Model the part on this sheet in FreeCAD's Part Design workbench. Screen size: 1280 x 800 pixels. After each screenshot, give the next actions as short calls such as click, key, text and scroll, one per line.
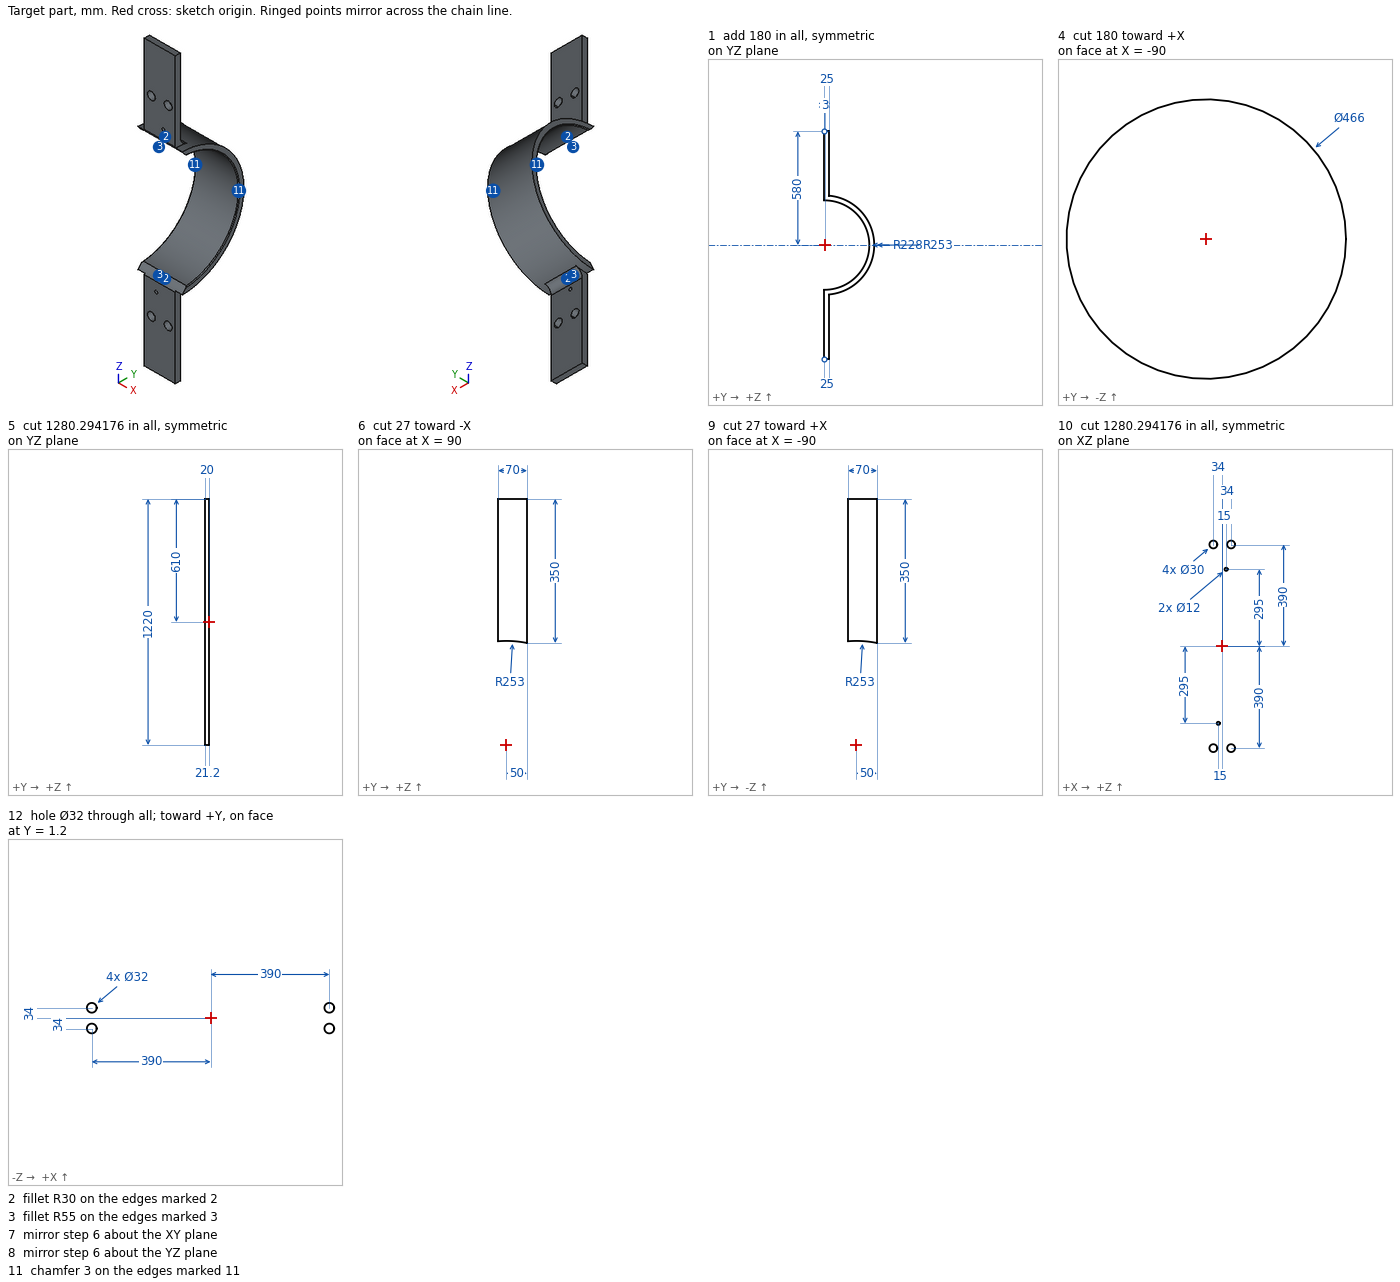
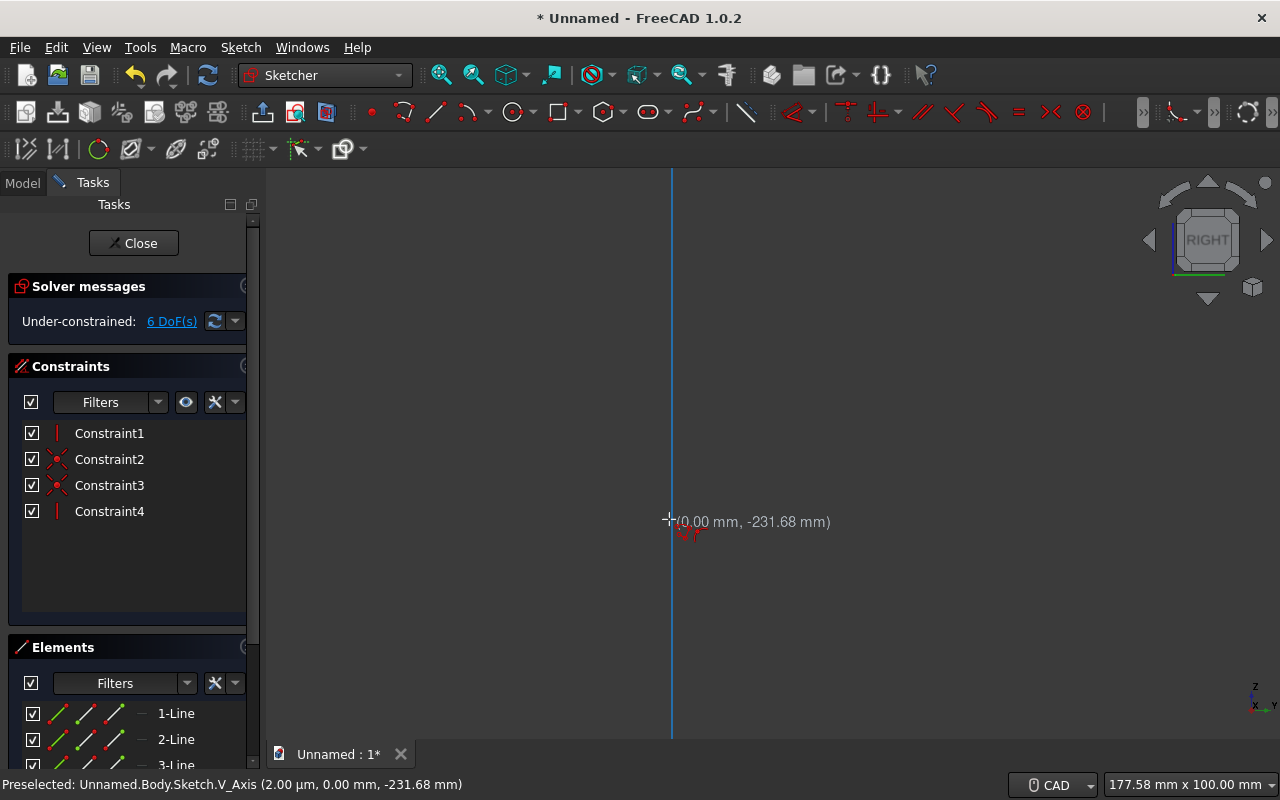
click(655, 506)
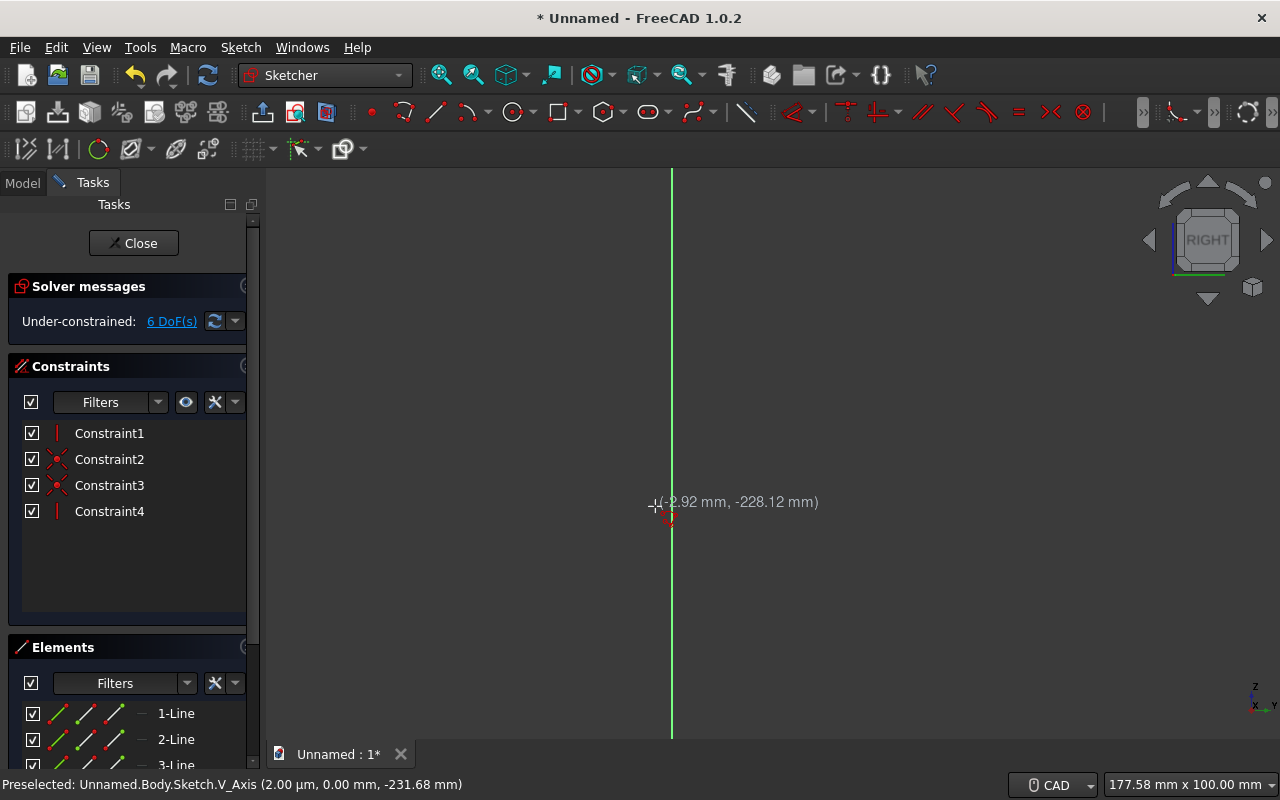
scroll(669, 519, down, 15)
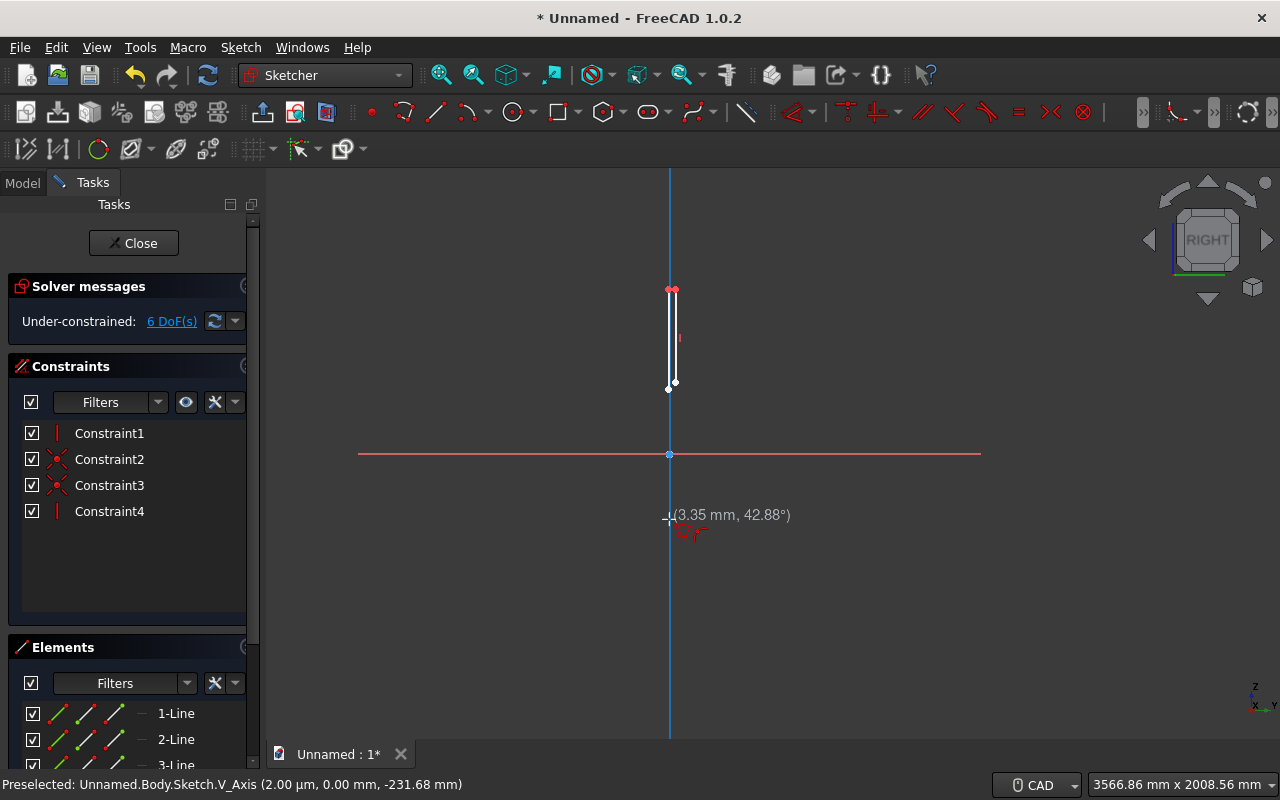
scroll(669, 619, up, 15)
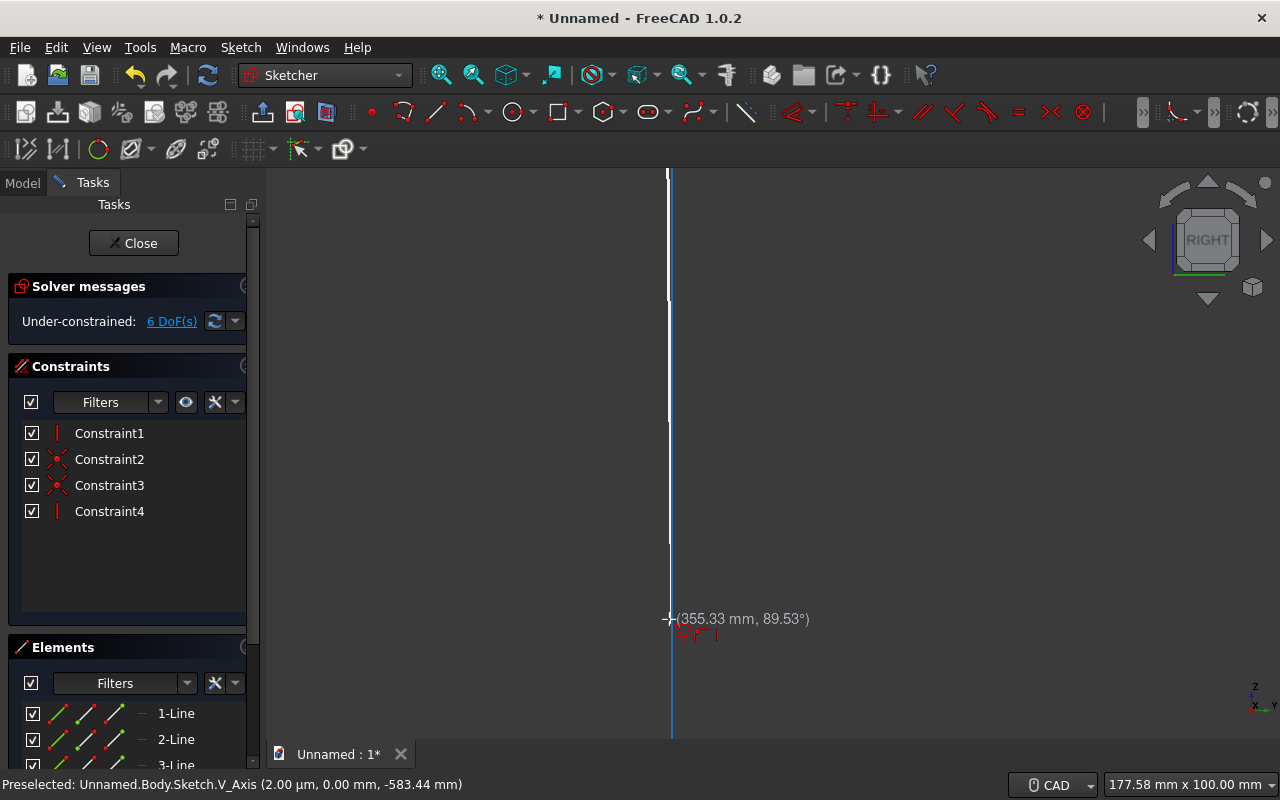
click(655, 604)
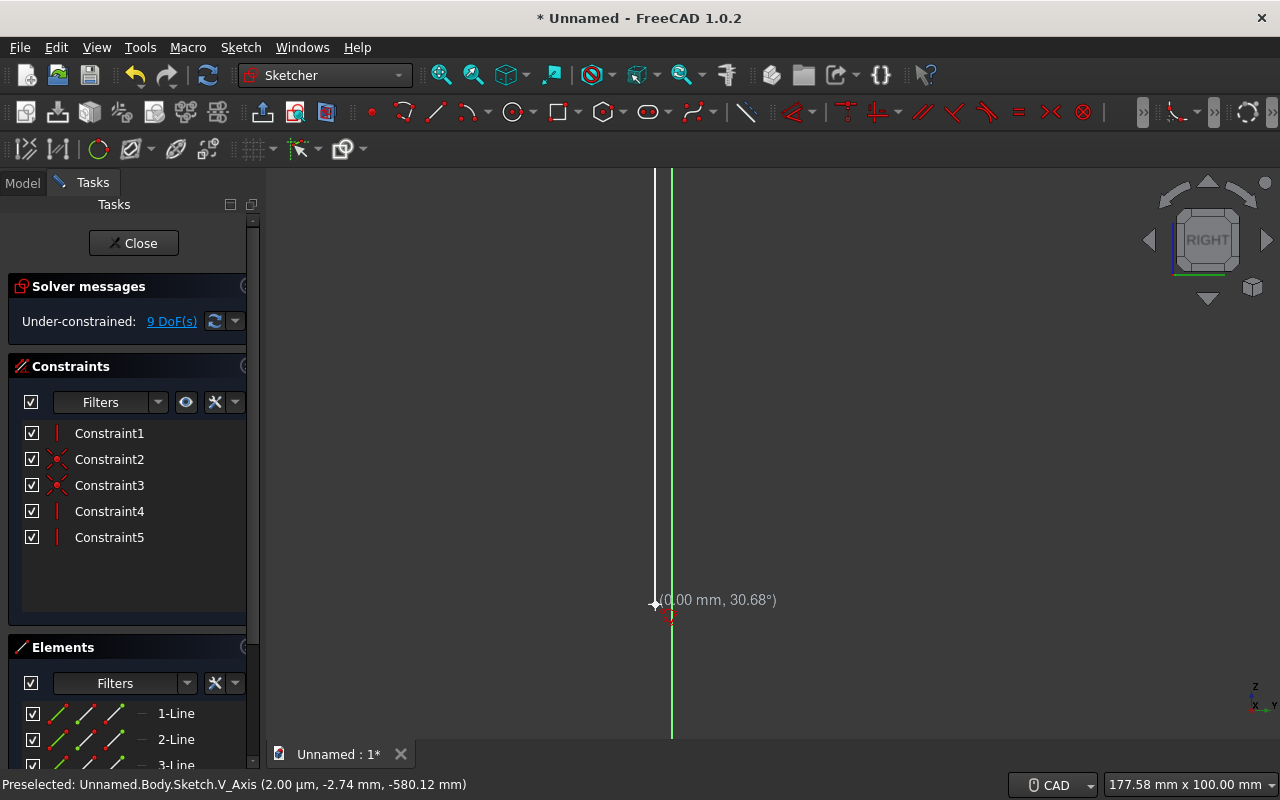
scroll(669, 619, down, 15)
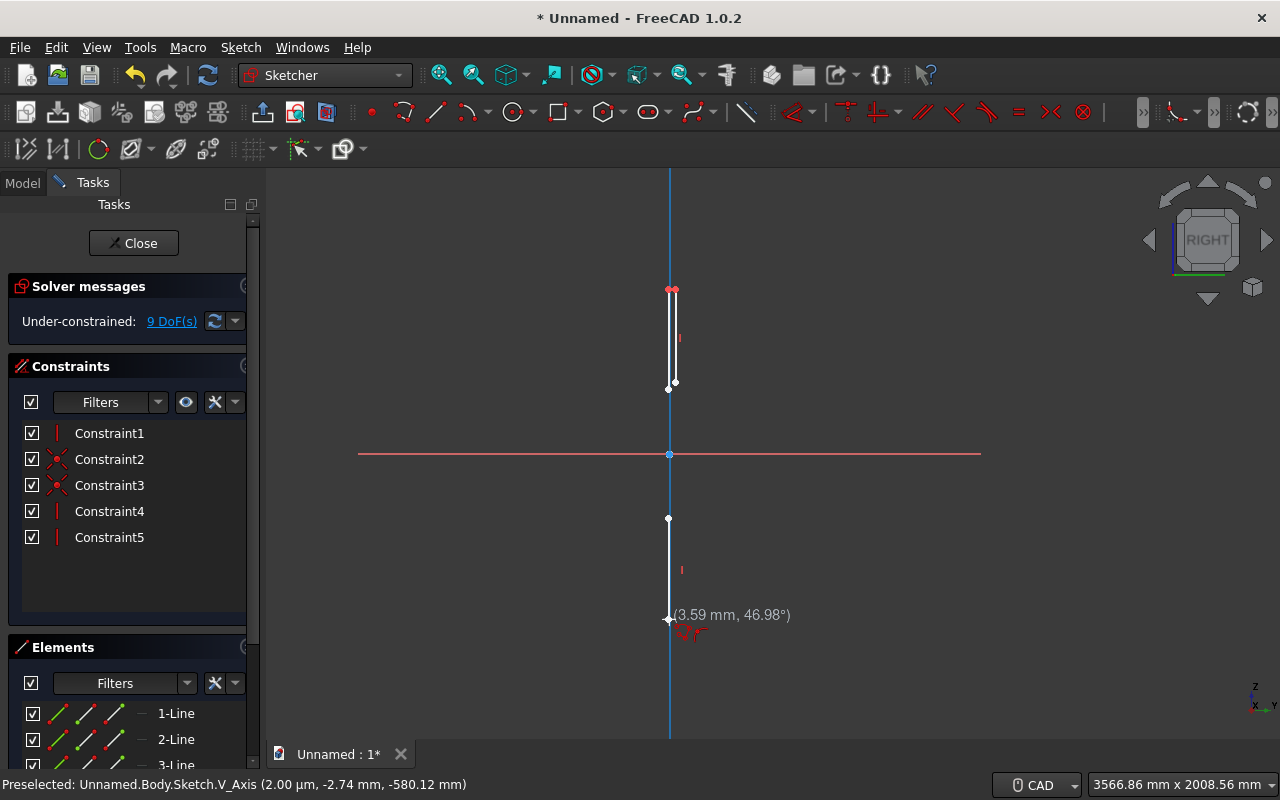
scroll(676, 619, up, 5)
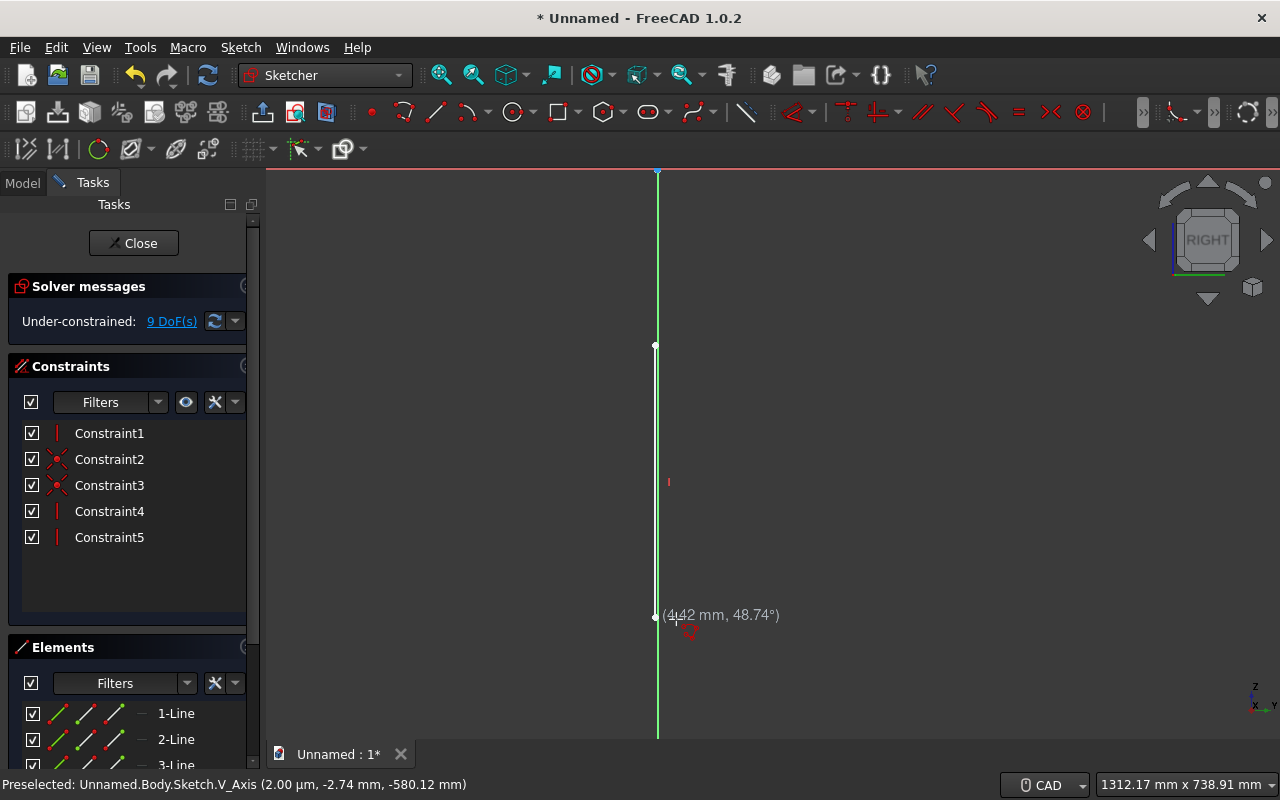
click(675, 618)
click(675, 364)
right_click(675, 364)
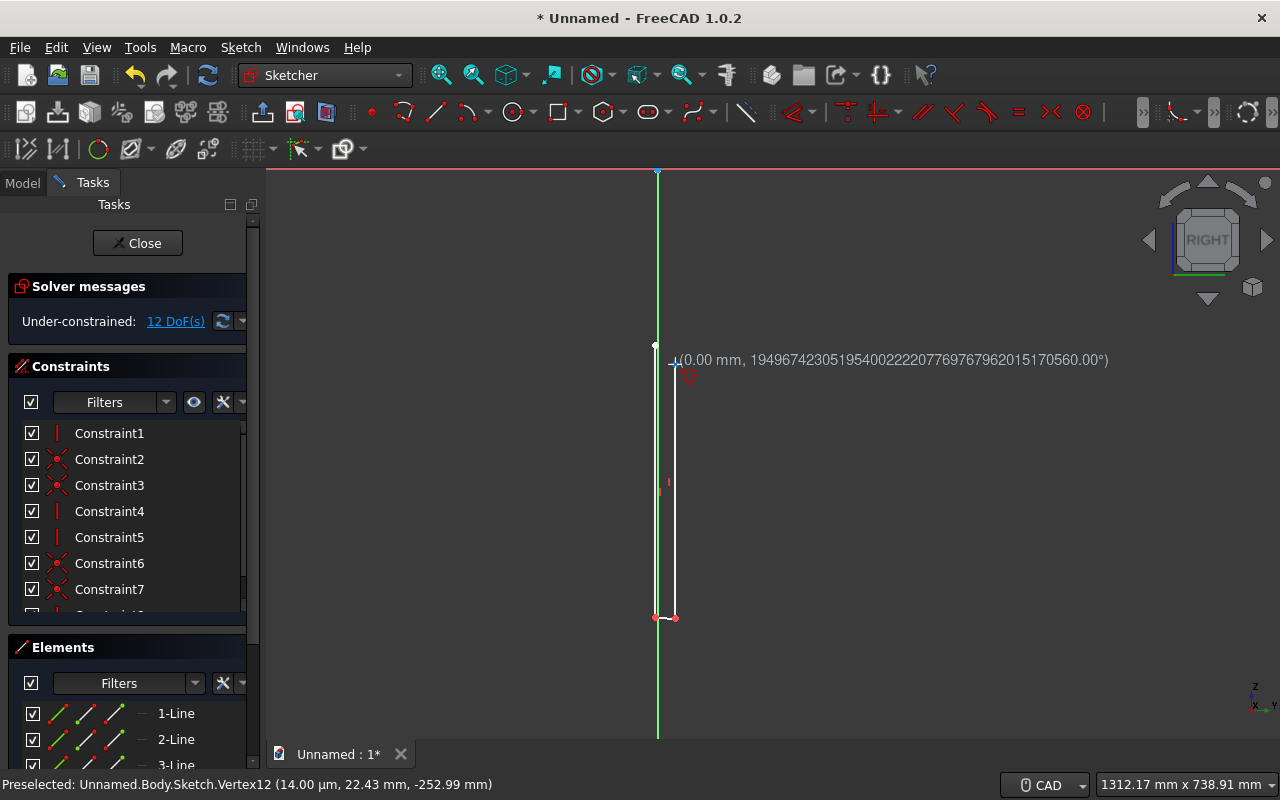
click(490, 112)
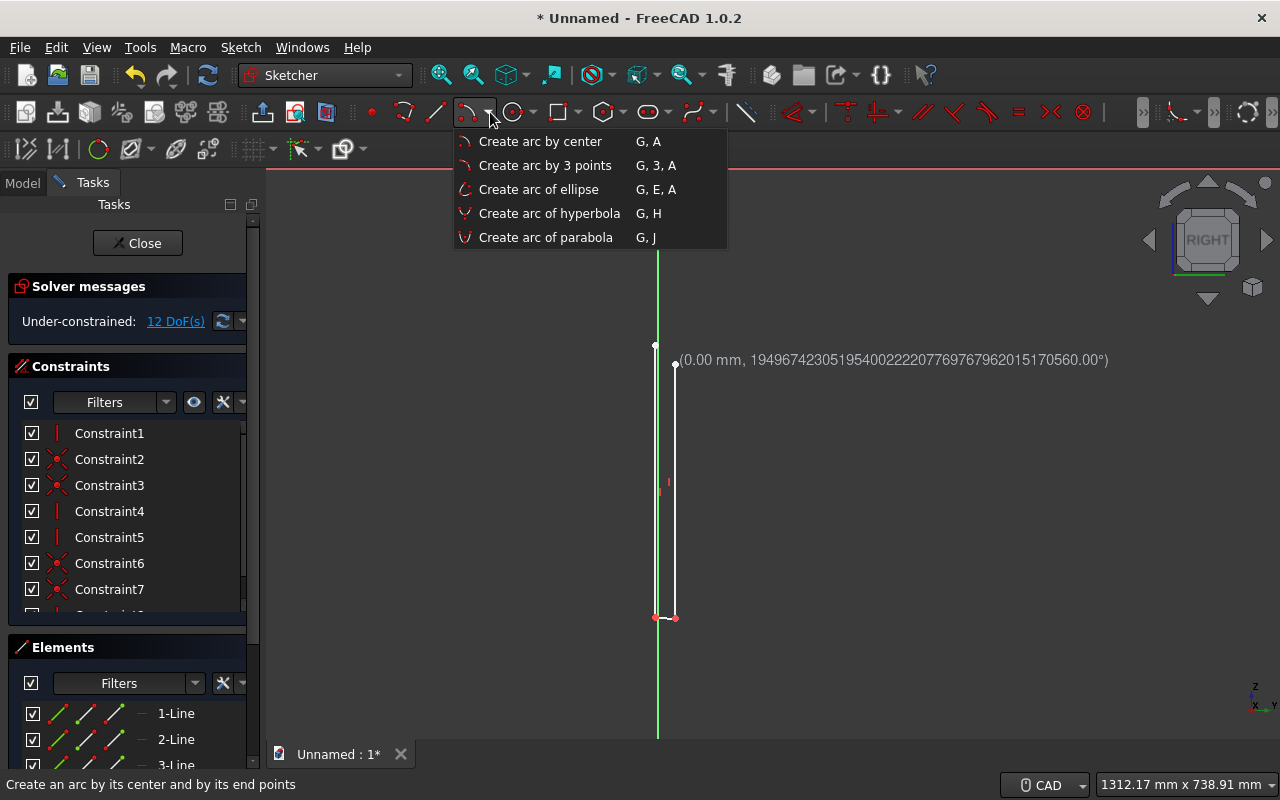
click(590, 165)